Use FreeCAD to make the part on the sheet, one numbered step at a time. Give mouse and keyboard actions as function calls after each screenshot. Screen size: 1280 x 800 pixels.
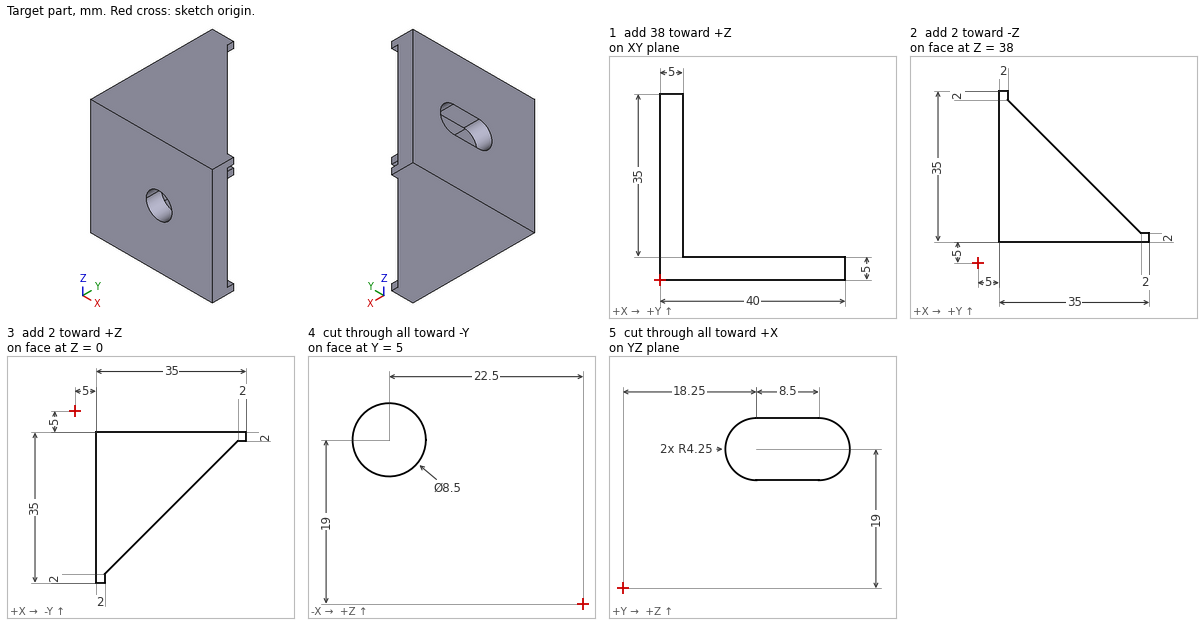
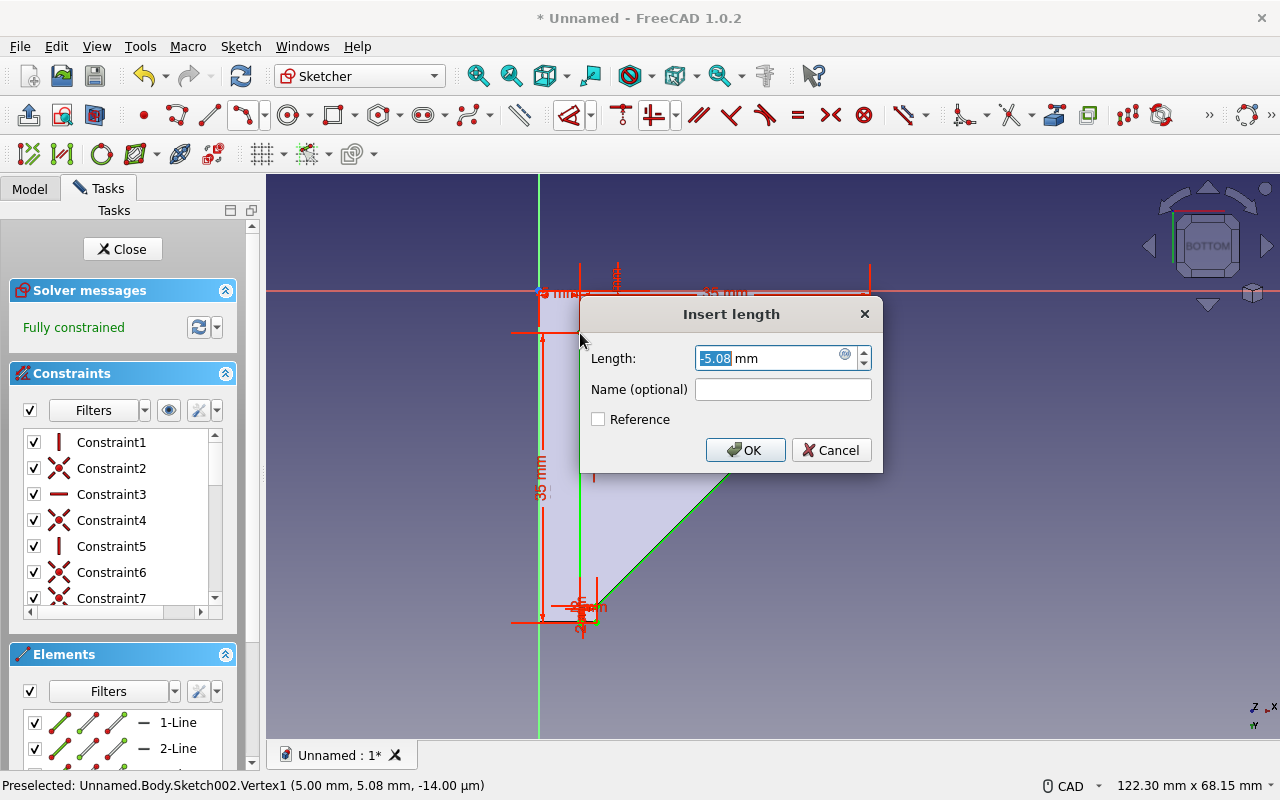
text(-5)
key(Return)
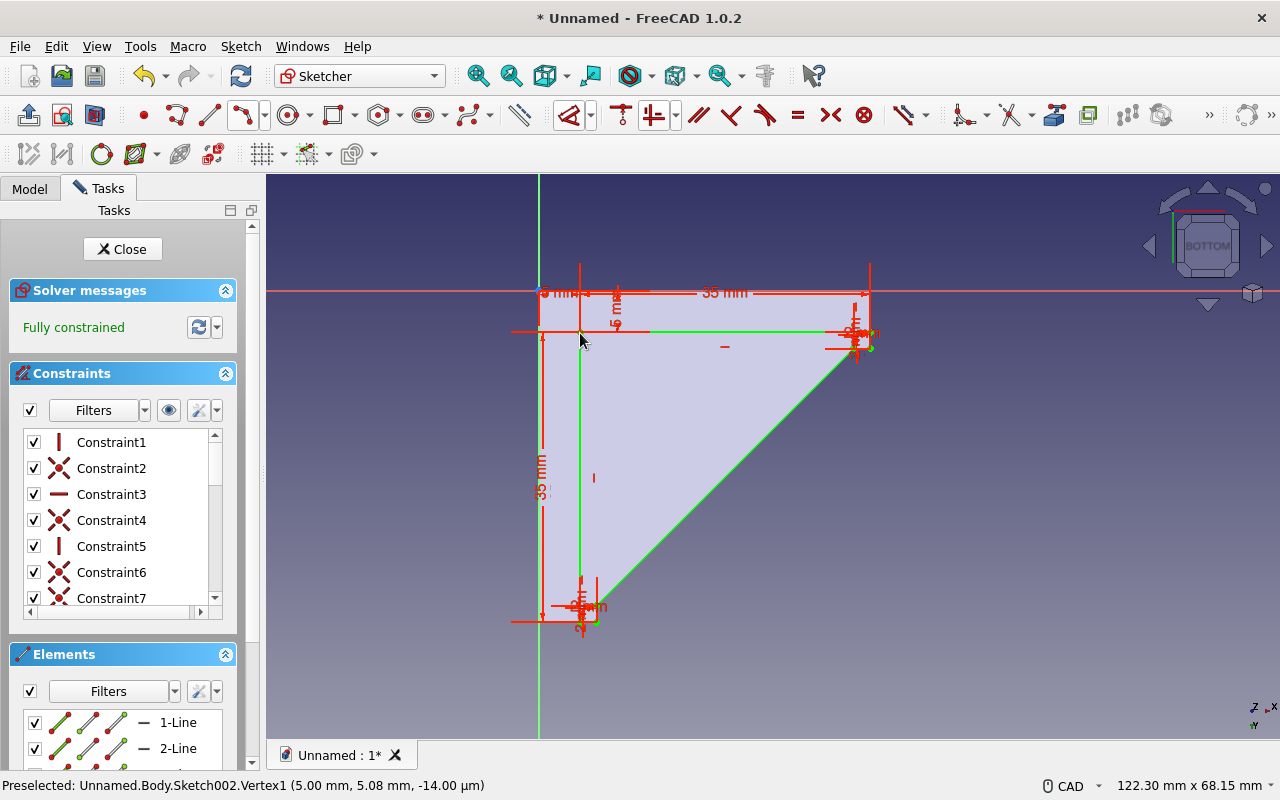
click(123, 249)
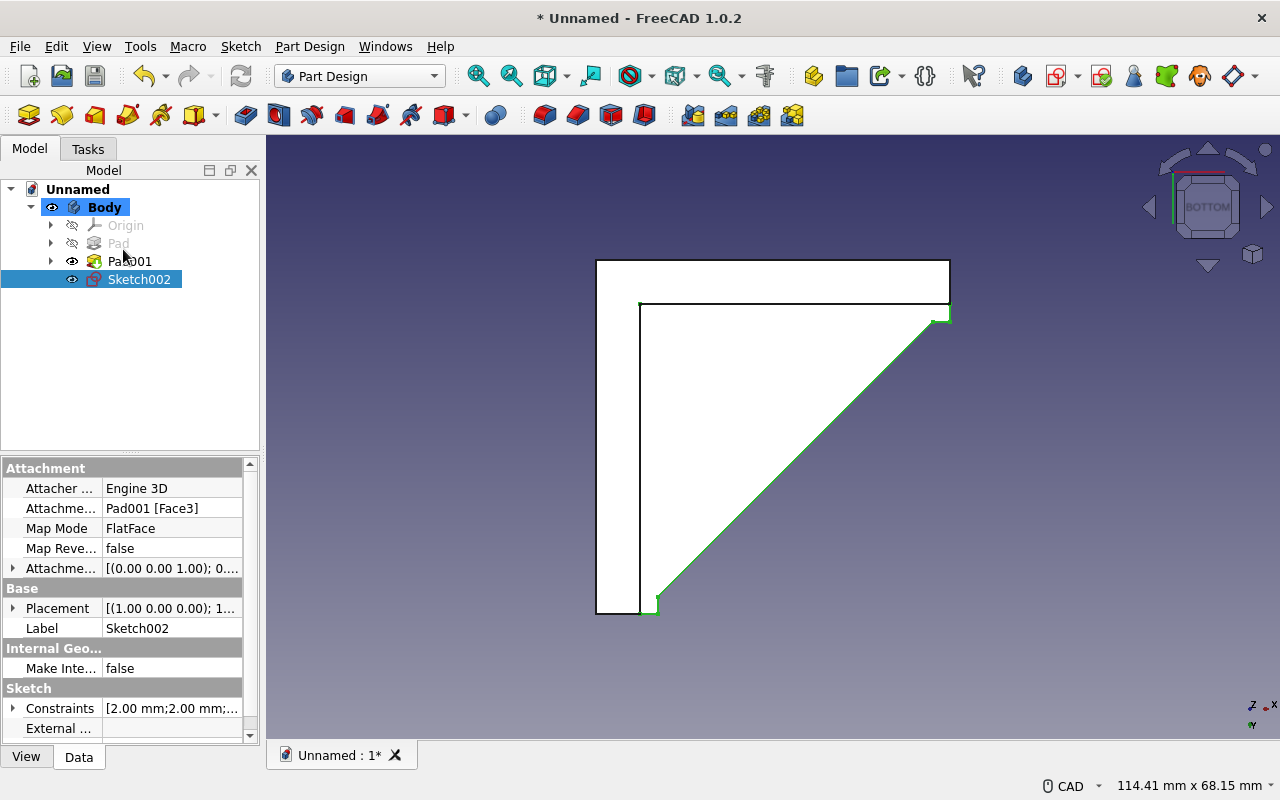
click(29, 116)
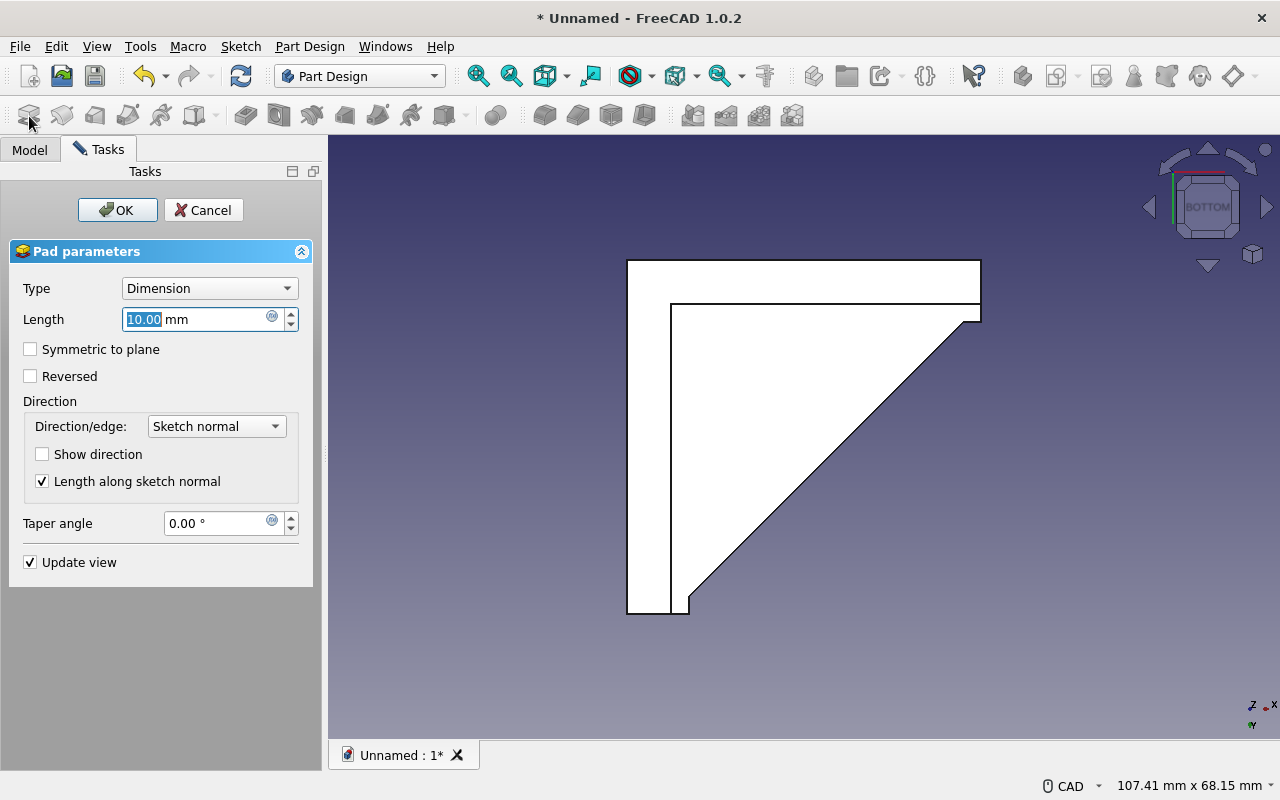
text(2)
key(Tab)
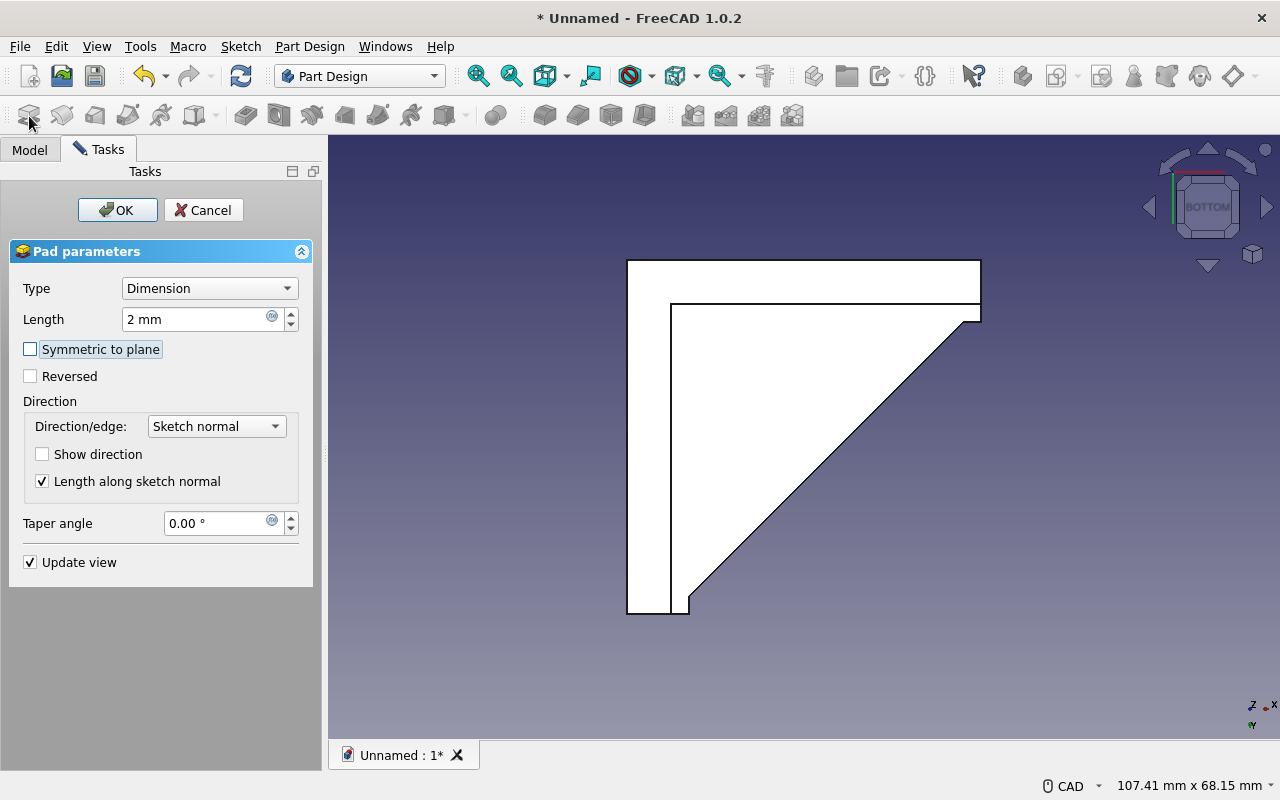
click(31, 376)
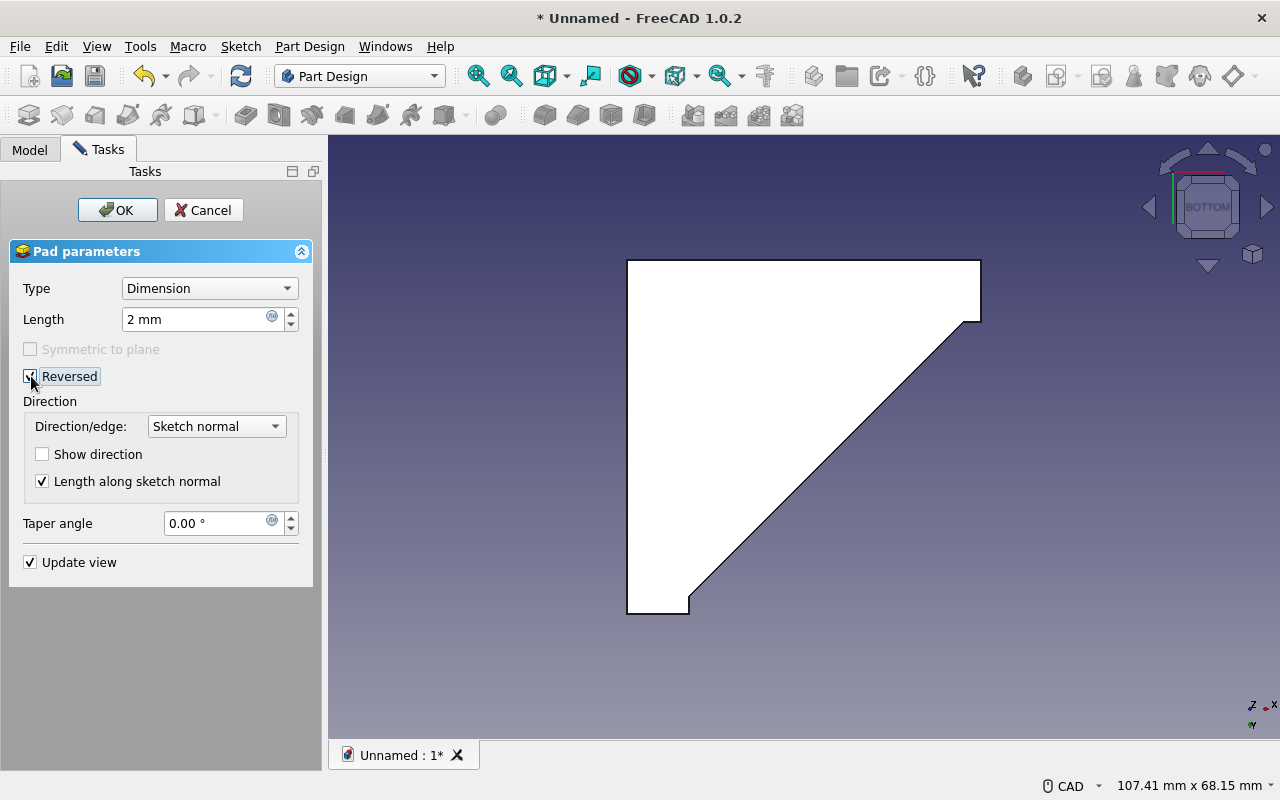
click(118, 210)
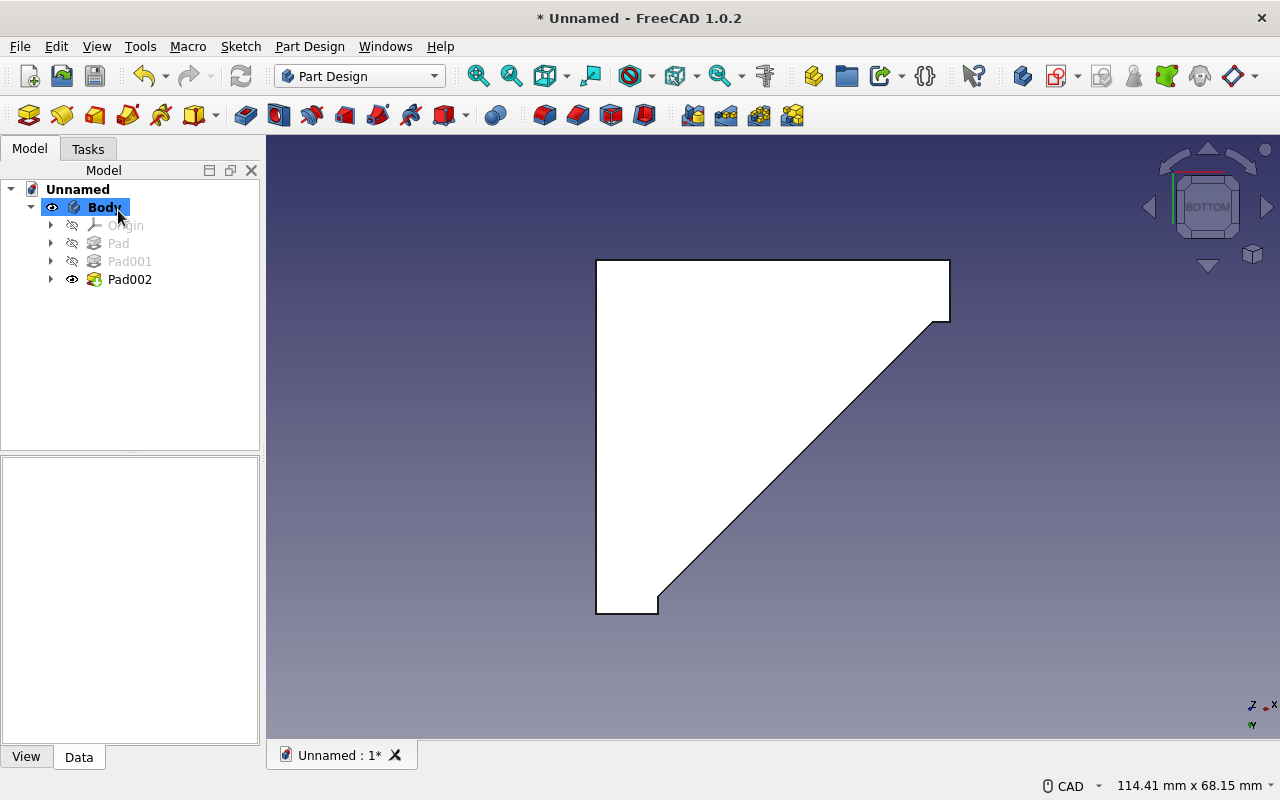
key(4)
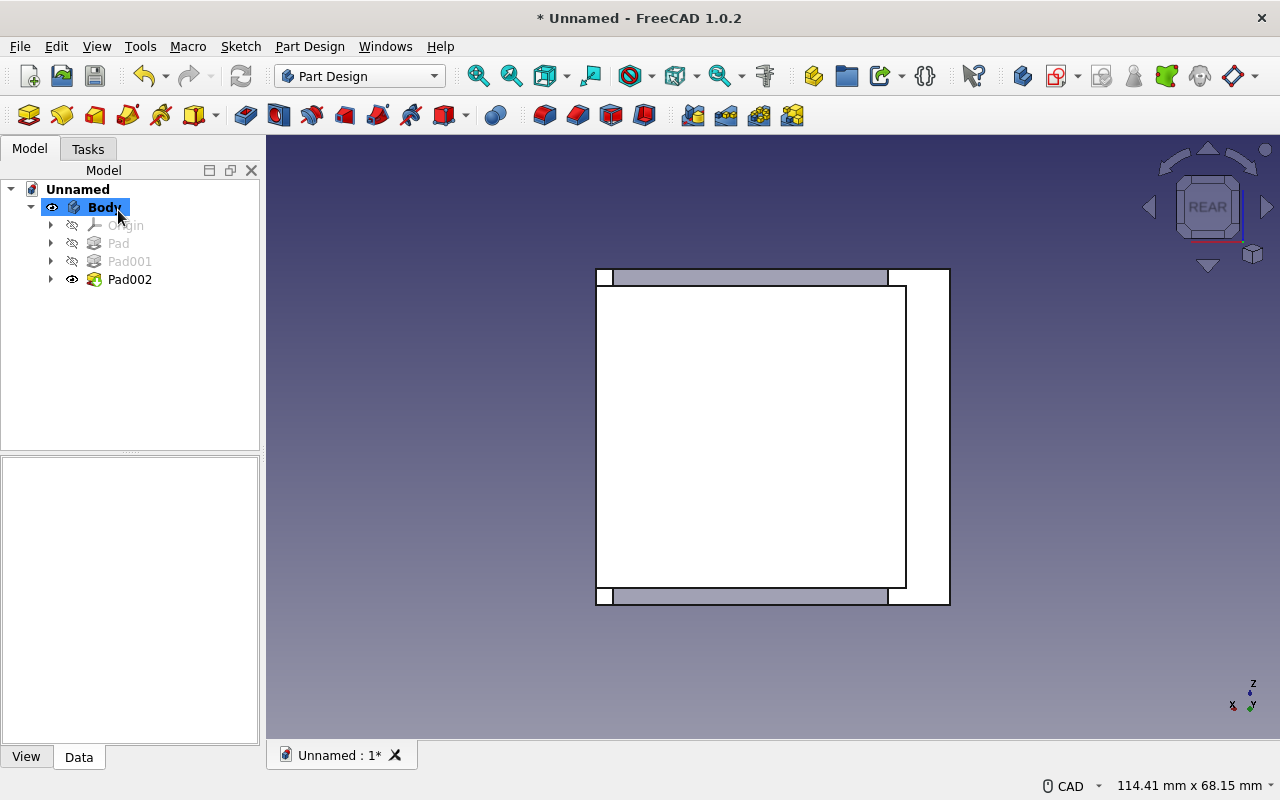
click(751, 436)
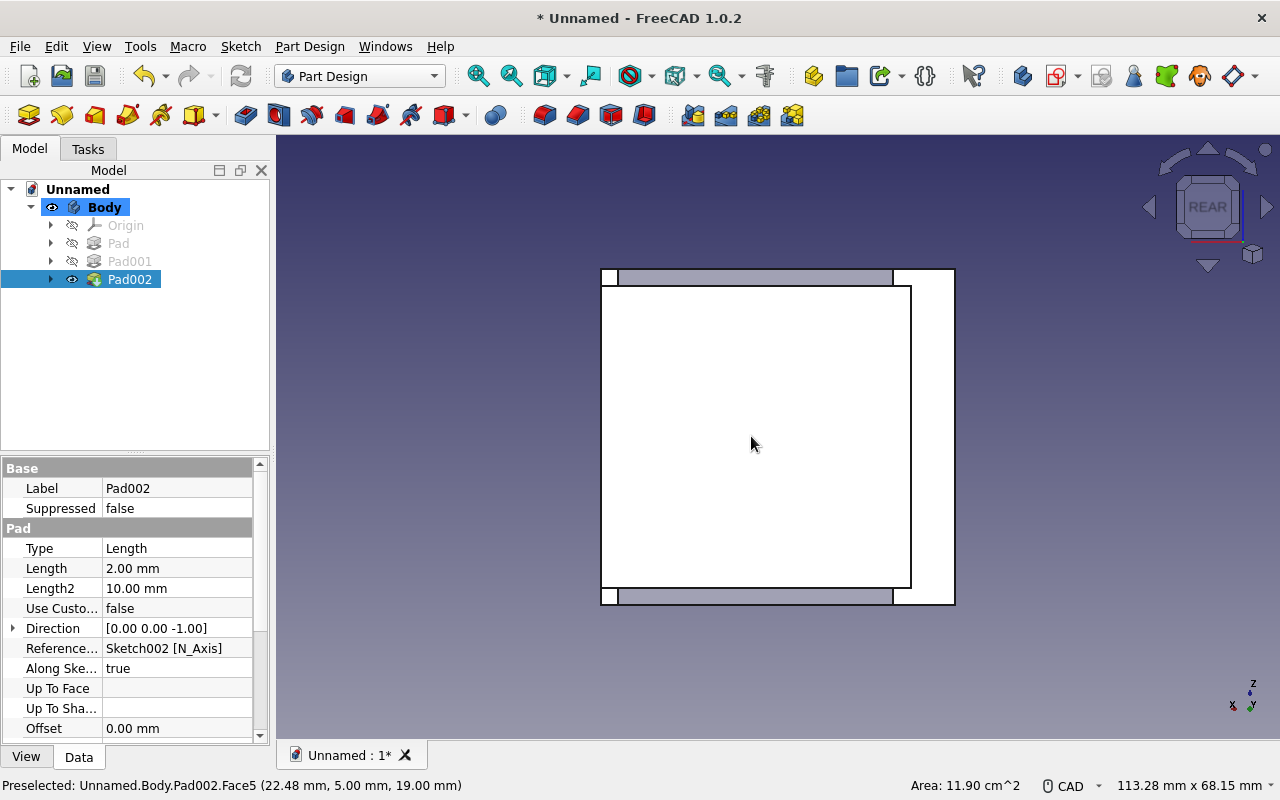
click(1056, 76)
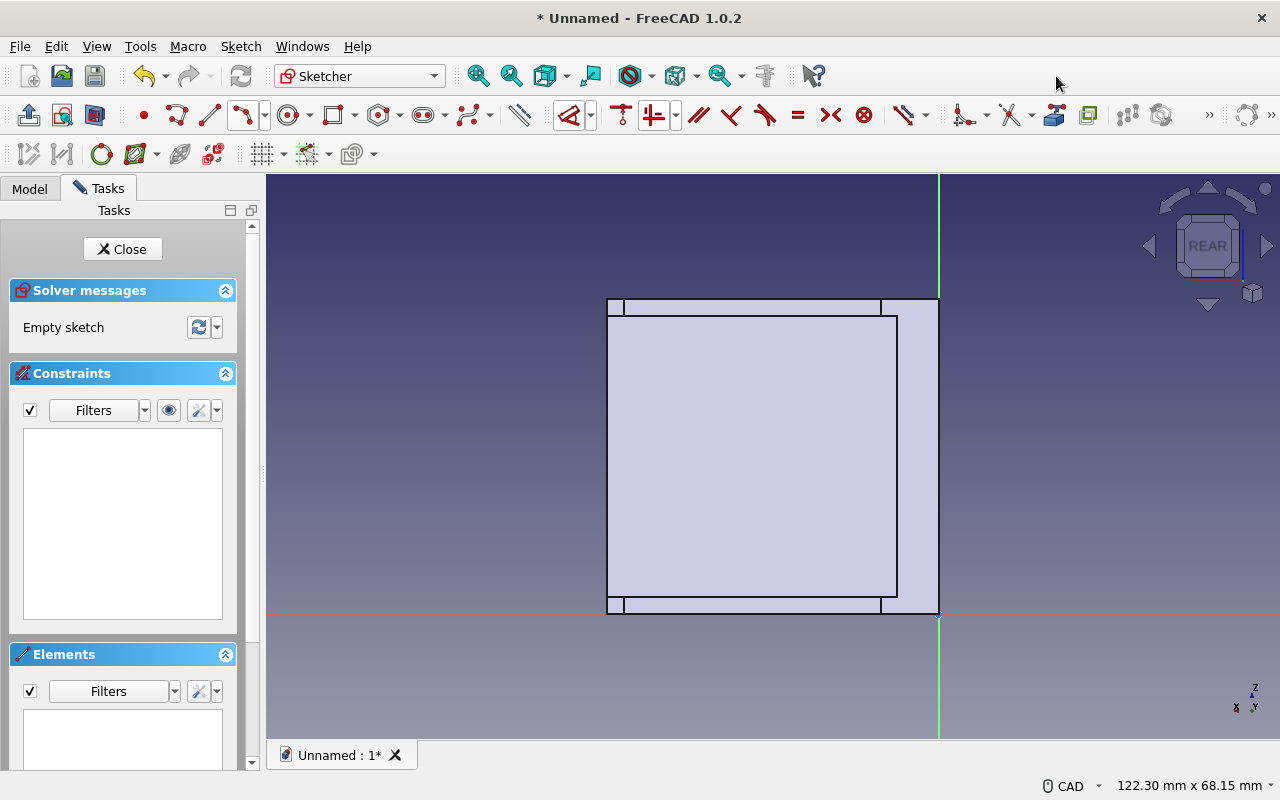
scroll(764, 457, up, 8)